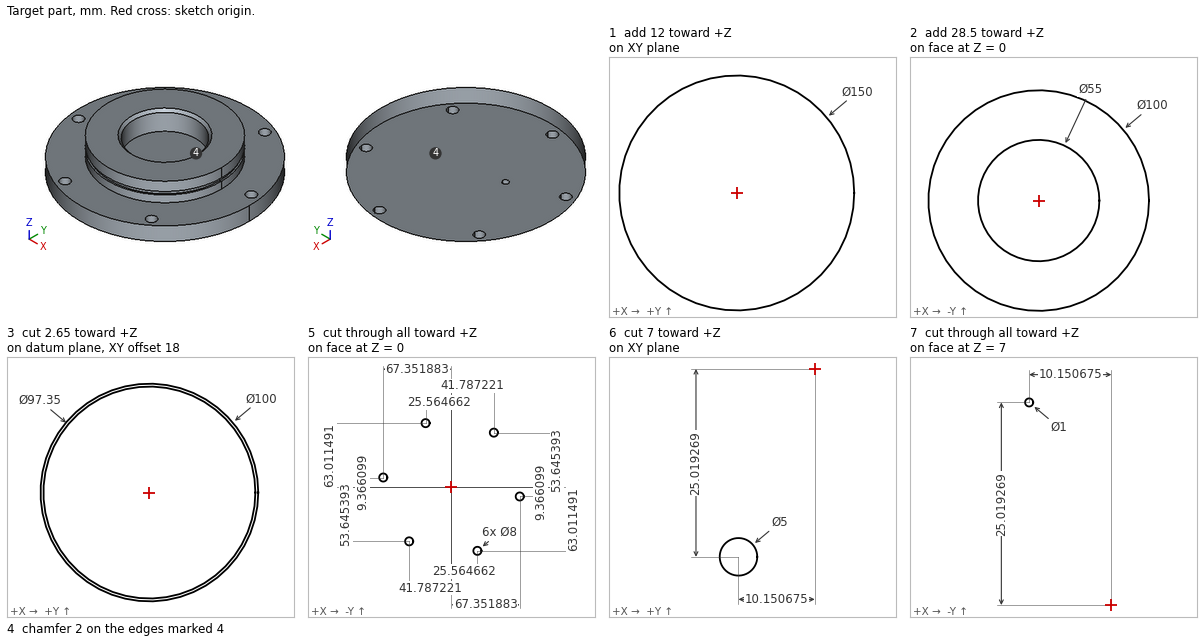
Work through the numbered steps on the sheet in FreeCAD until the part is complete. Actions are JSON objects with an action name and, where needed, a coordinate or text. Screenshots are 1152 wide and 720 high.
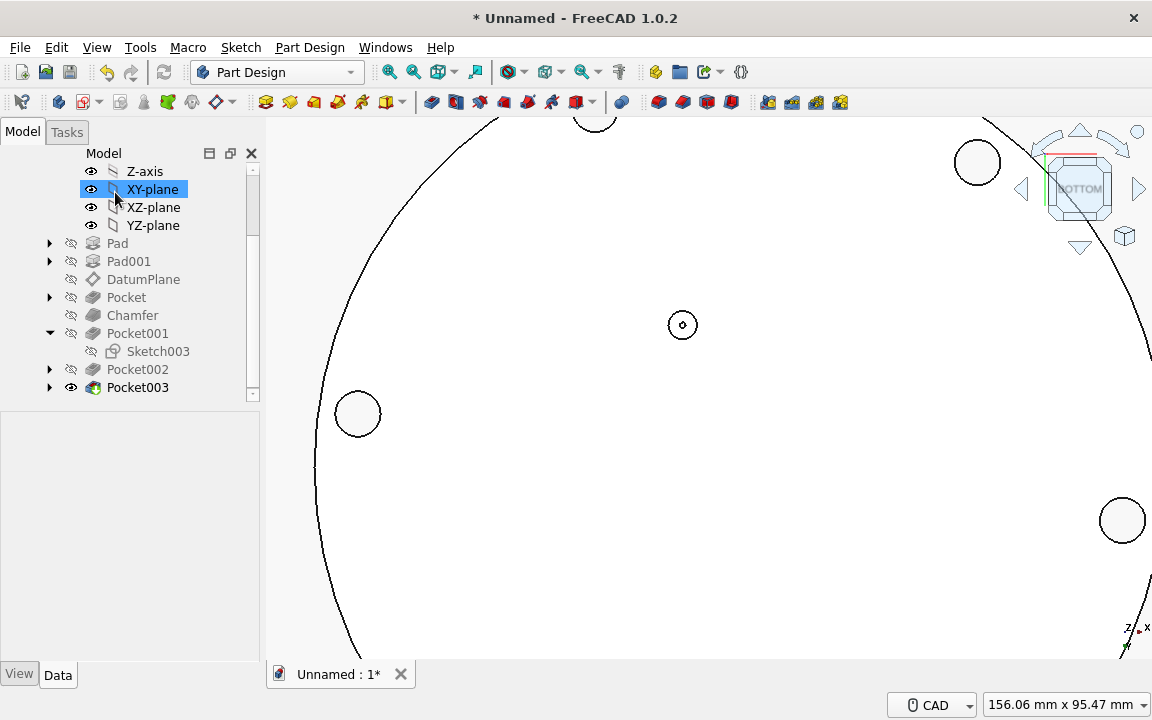
{"action": "key", "text": "0"}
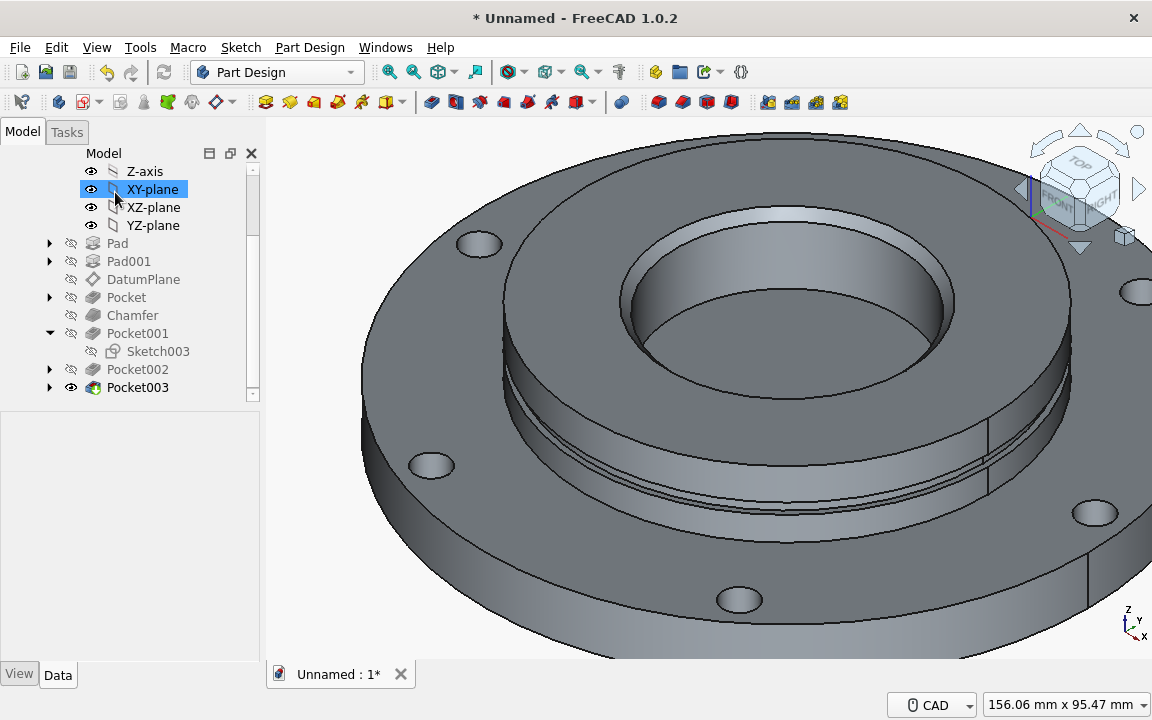
{"action": "left_click", "coordinate": [390, 72]}